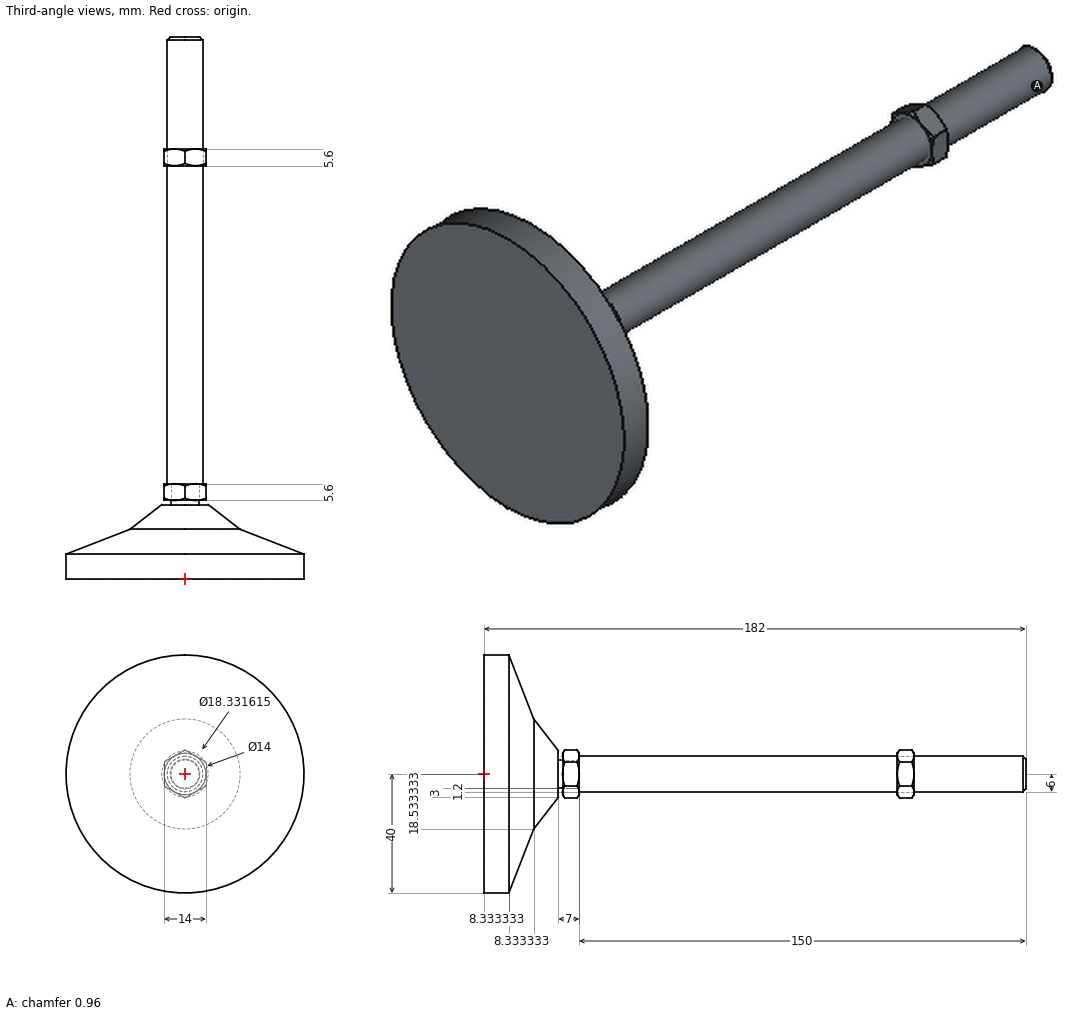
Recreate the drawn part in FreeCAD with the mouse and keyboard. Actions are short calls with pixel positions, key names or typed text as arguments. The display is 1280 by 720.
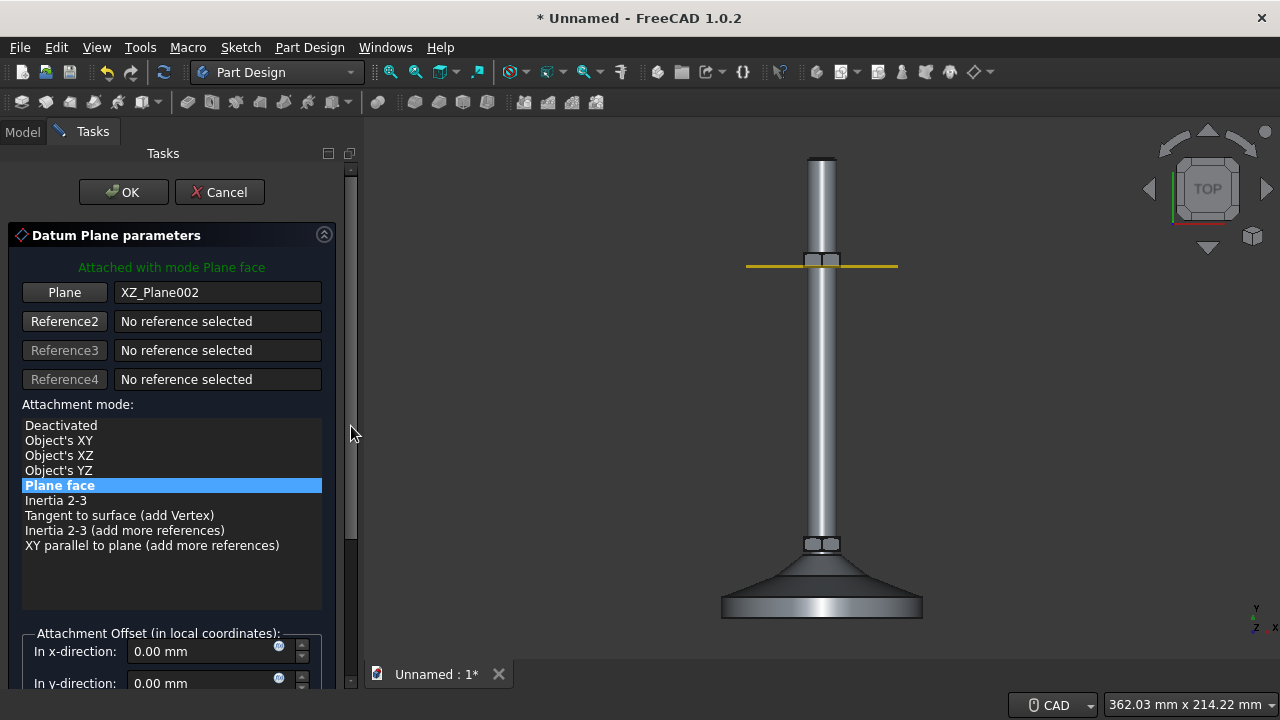
click(124, 192)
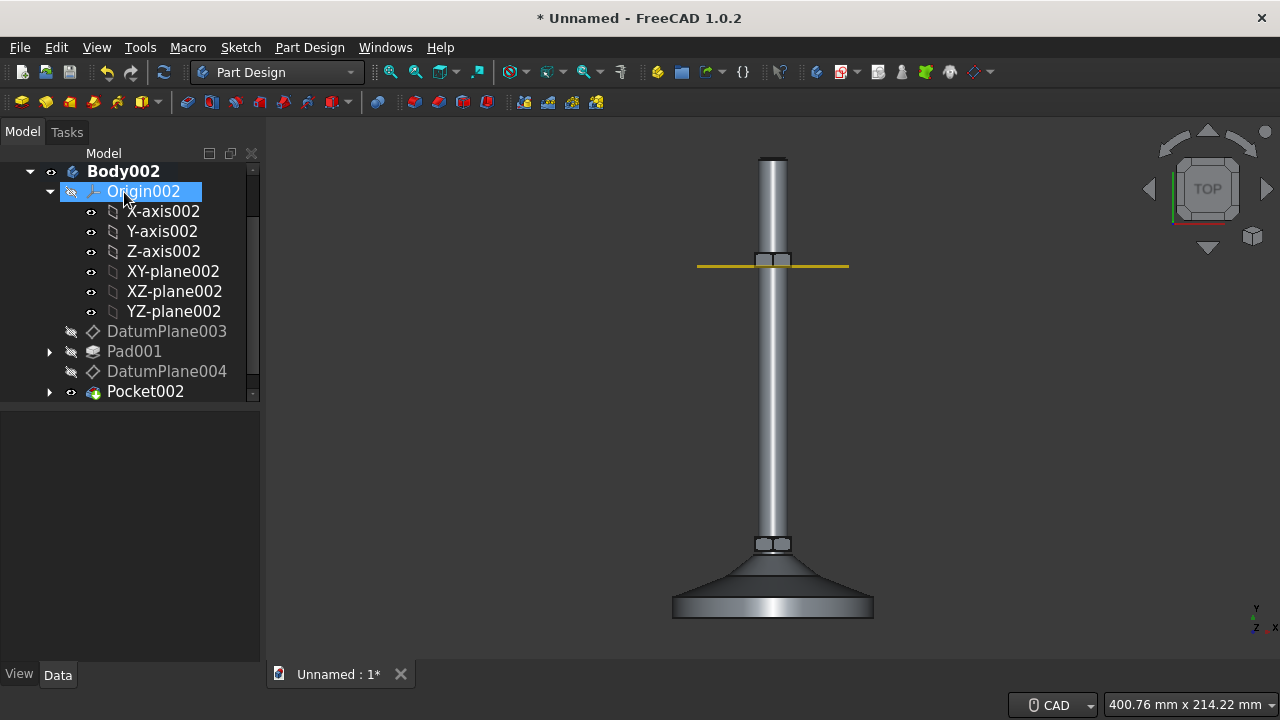
scroll(120, 287, down, 3)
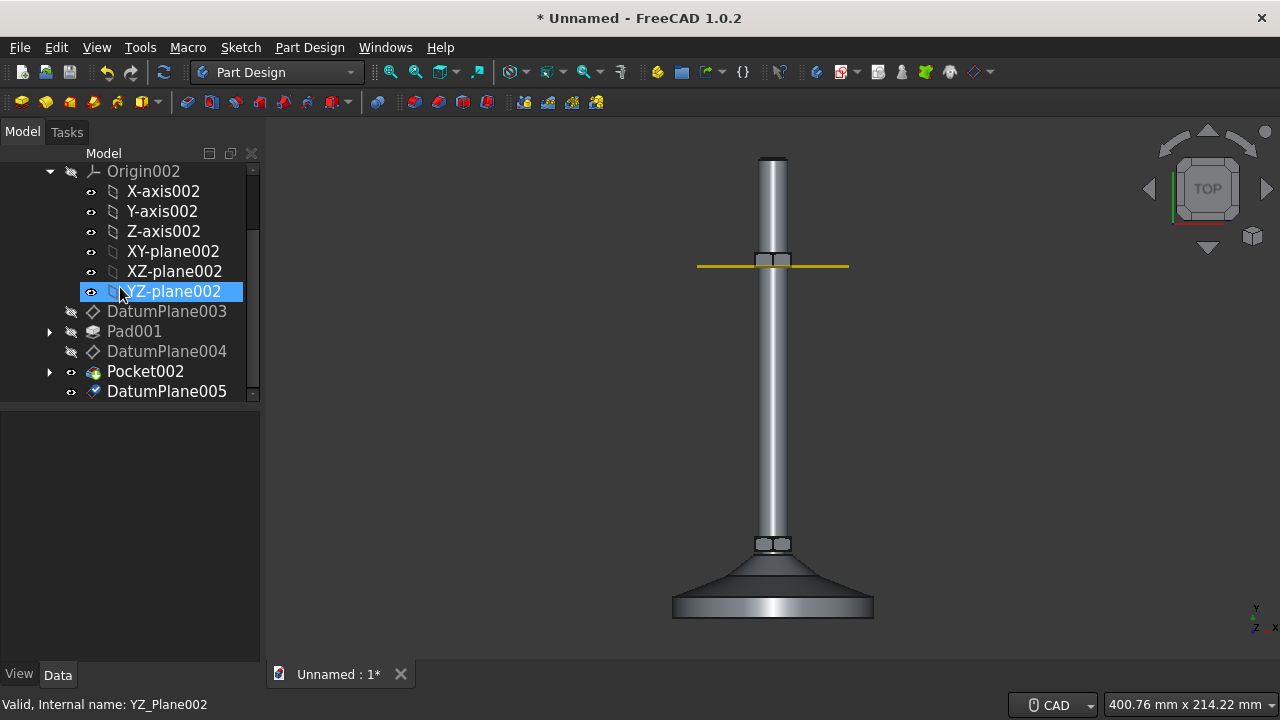
click(116, 392)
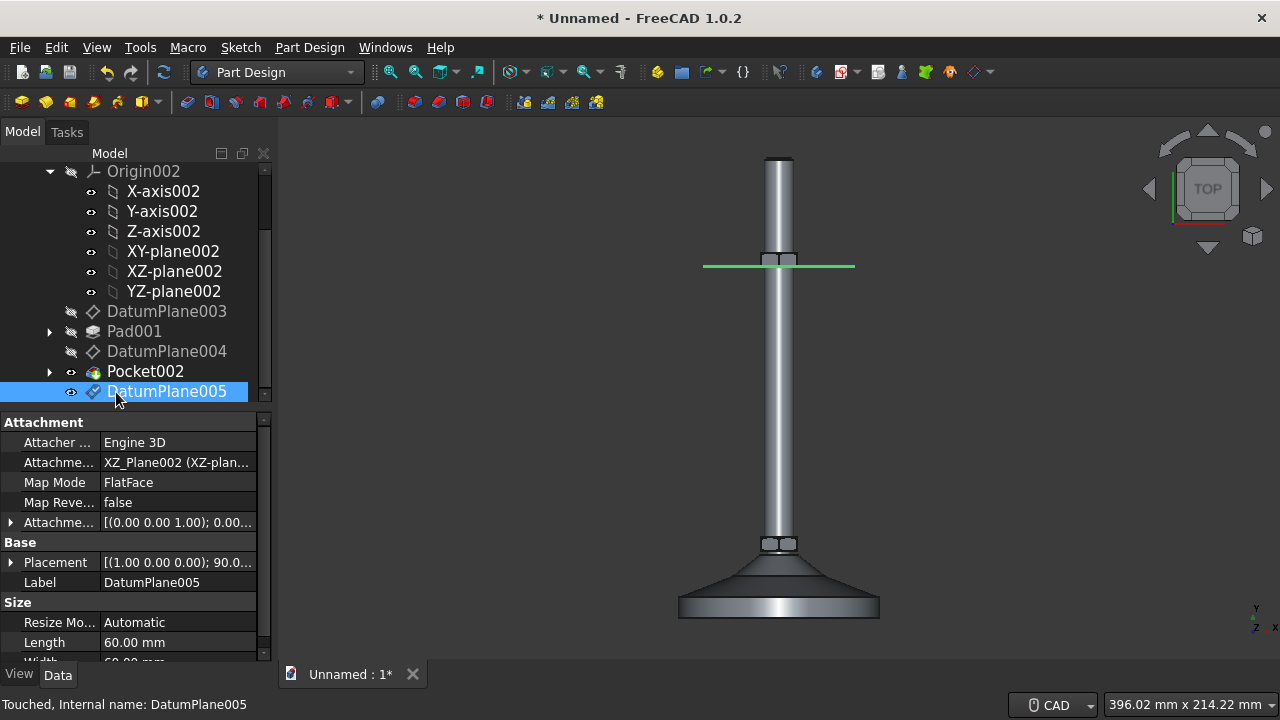
click(842, 72)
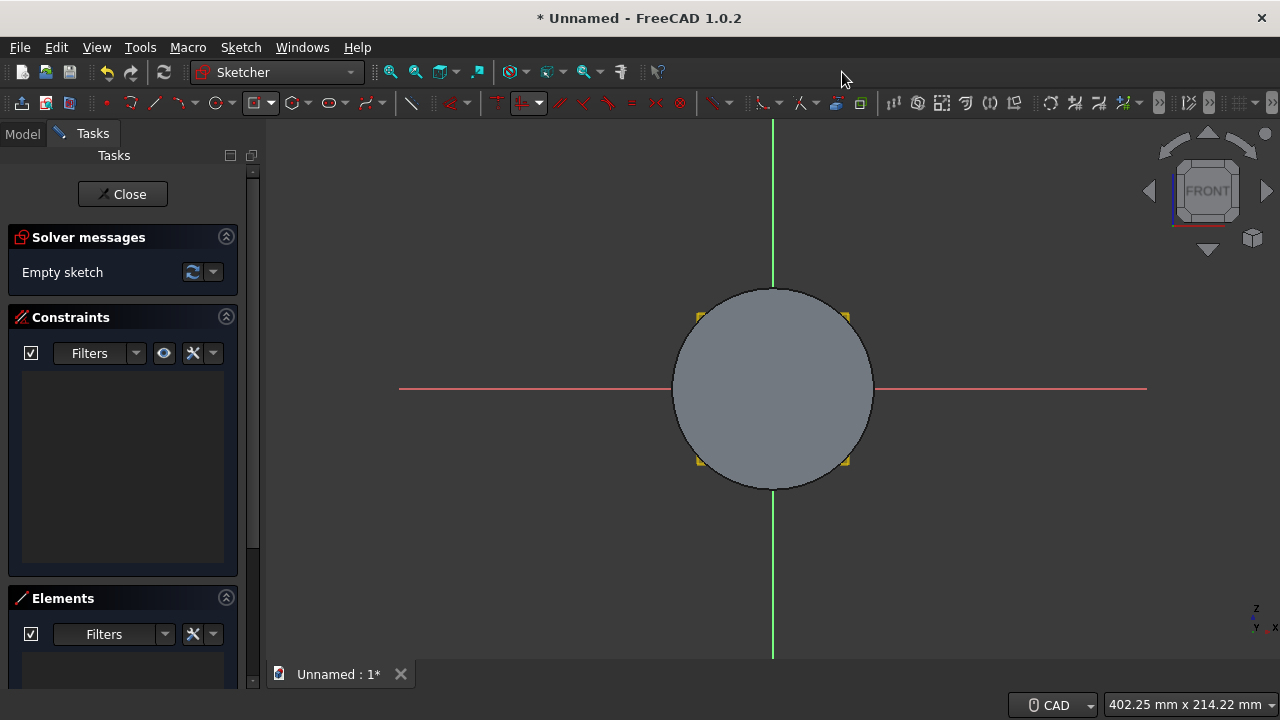
scroll(784, 389, up, 10)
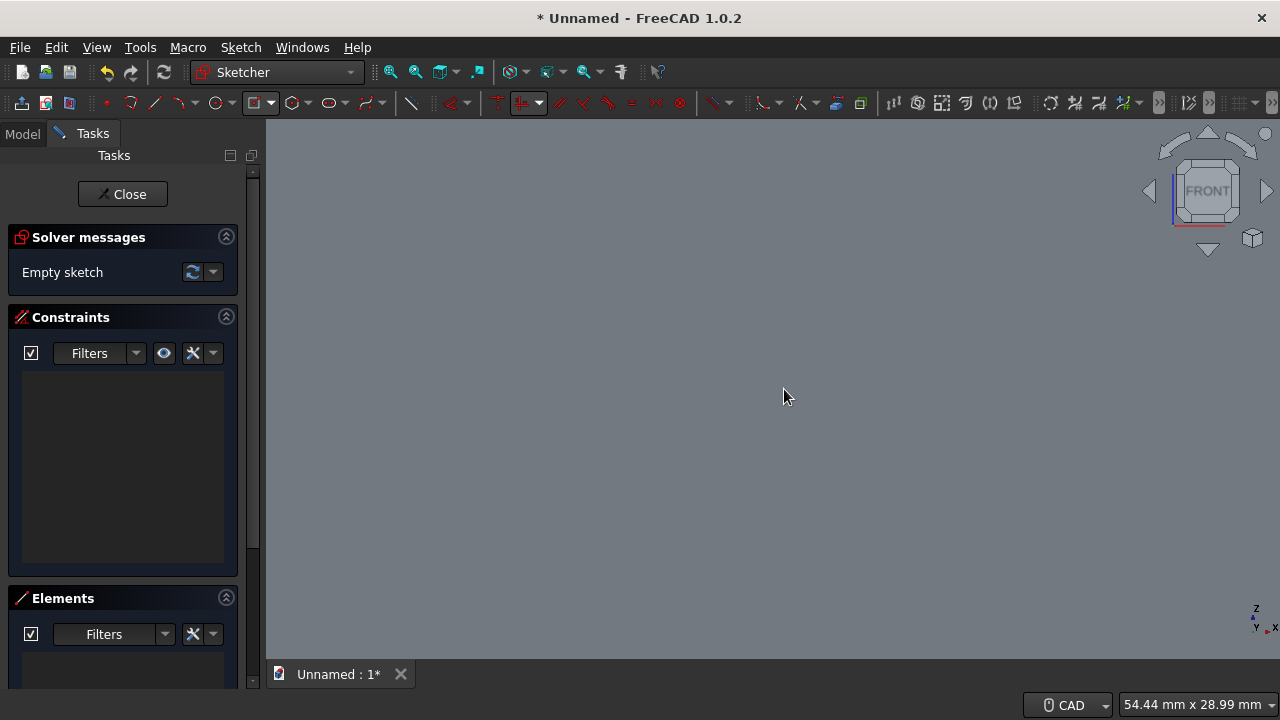
click(216, 104)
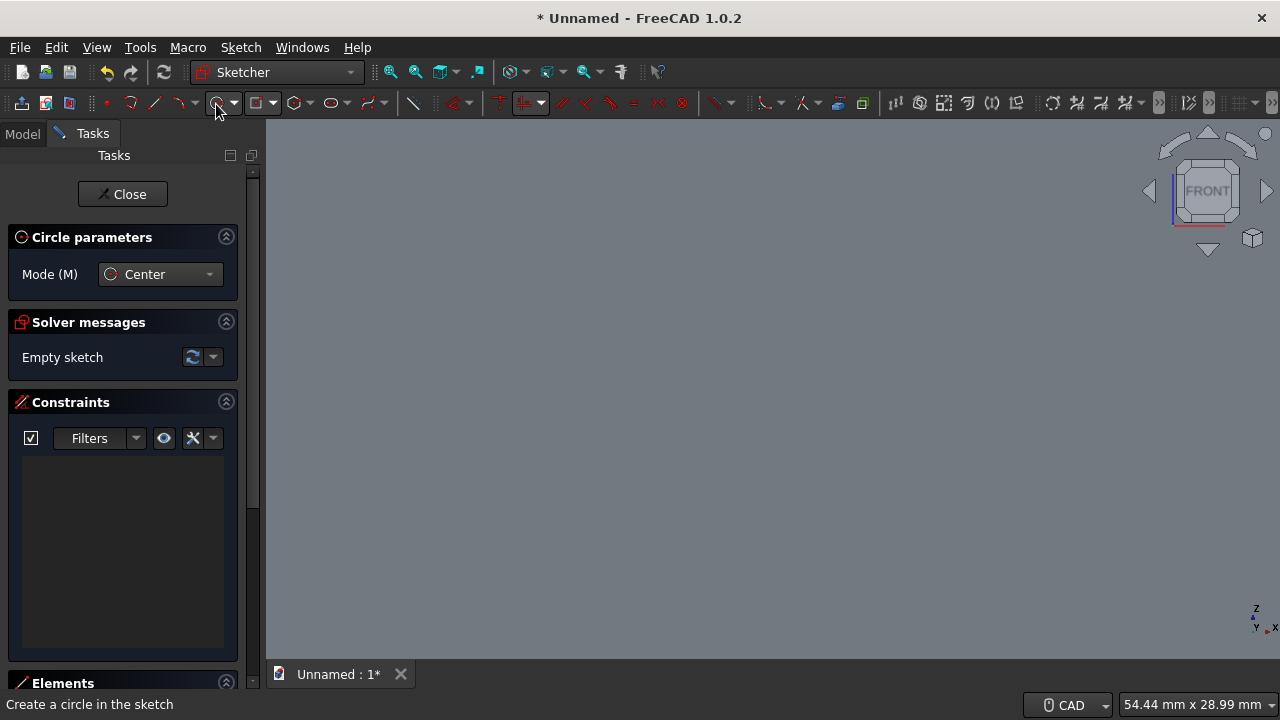
click(699, 386)
click(820, 265)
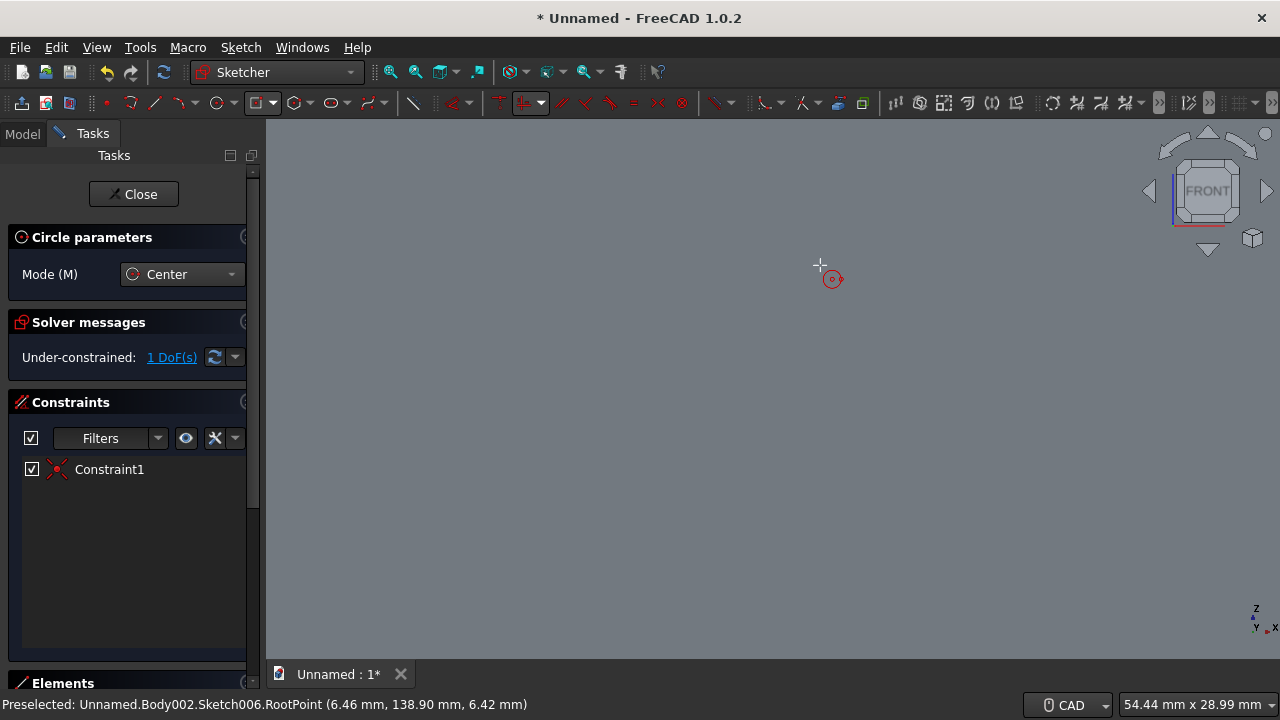
click(699, 386)
click(792, 294)
key(Escape)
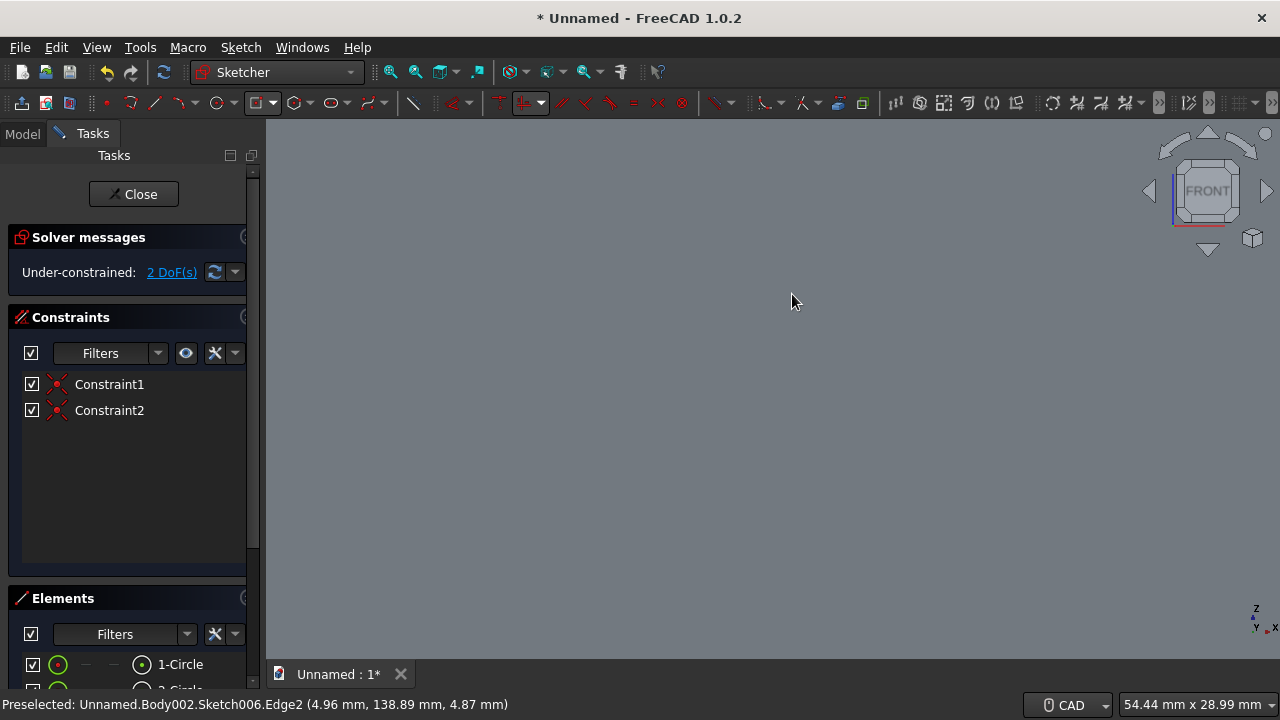
click(452, 104)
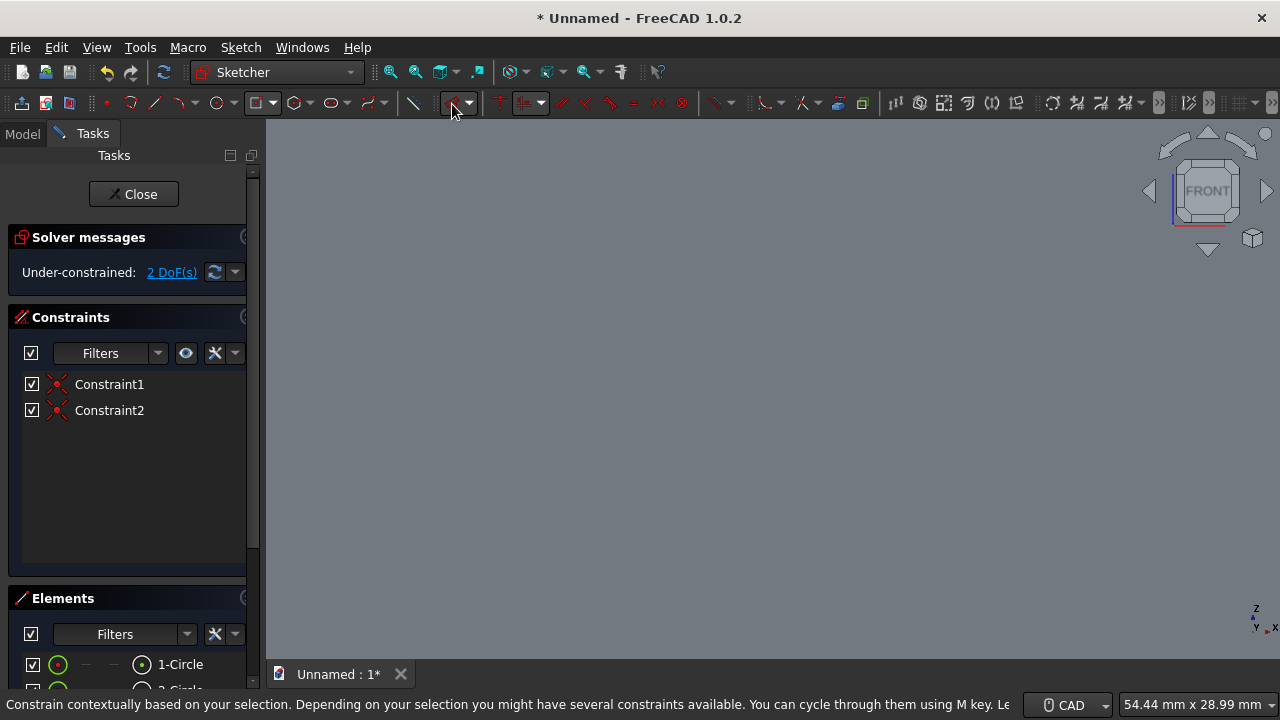
click(819, 265)
click(842, 242)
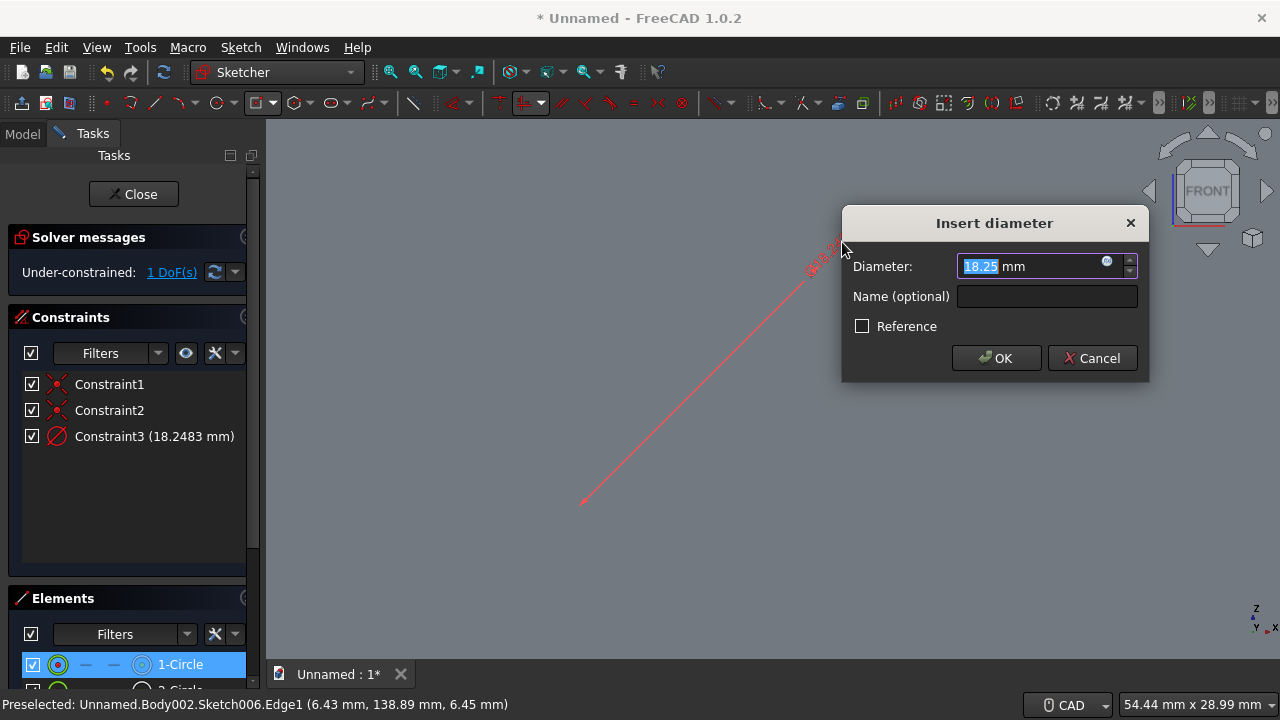
text(18.331615)
key(Return)